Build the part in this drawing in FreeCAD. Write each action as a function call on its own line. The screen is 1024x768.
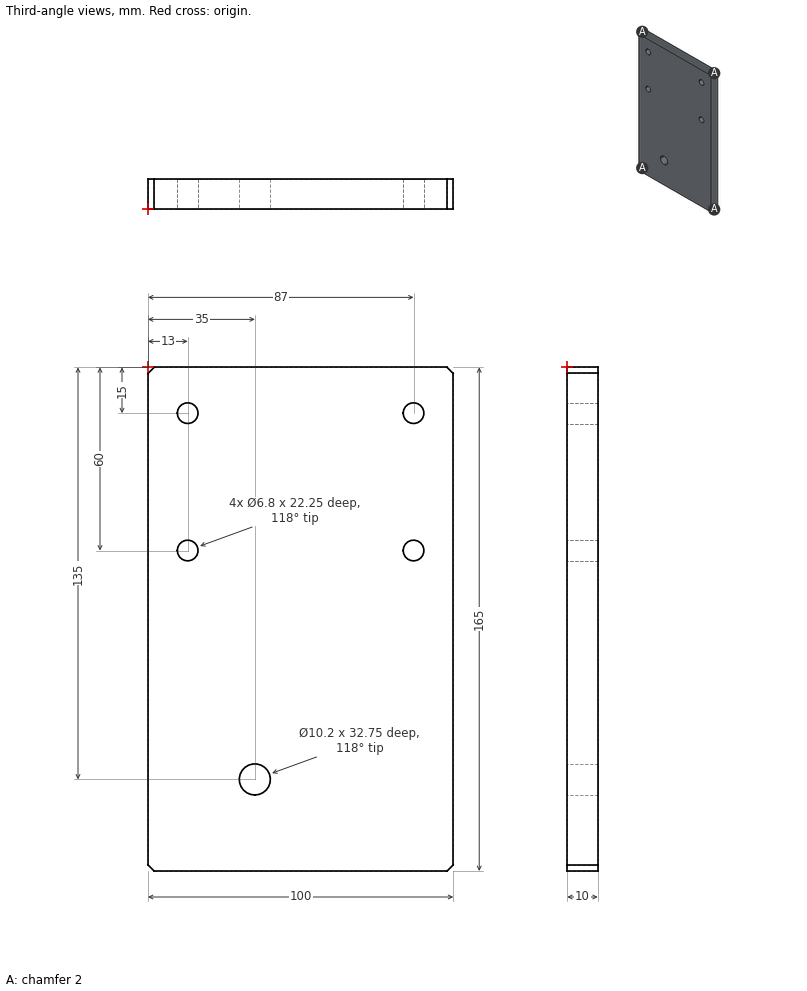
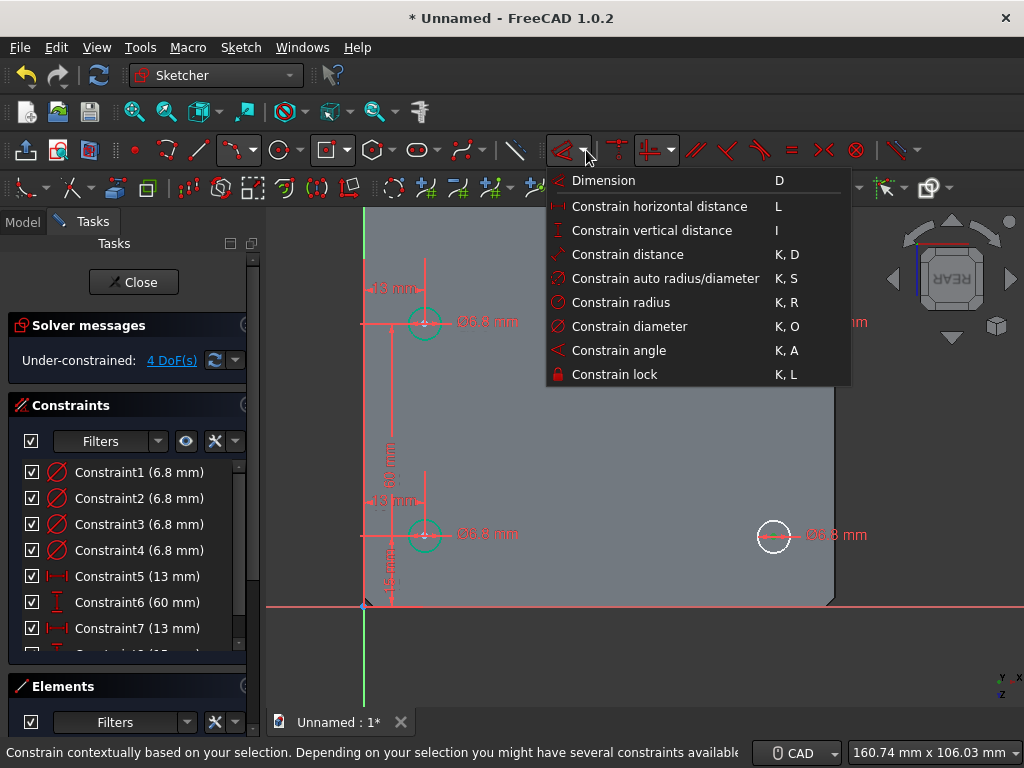
click(699, 206)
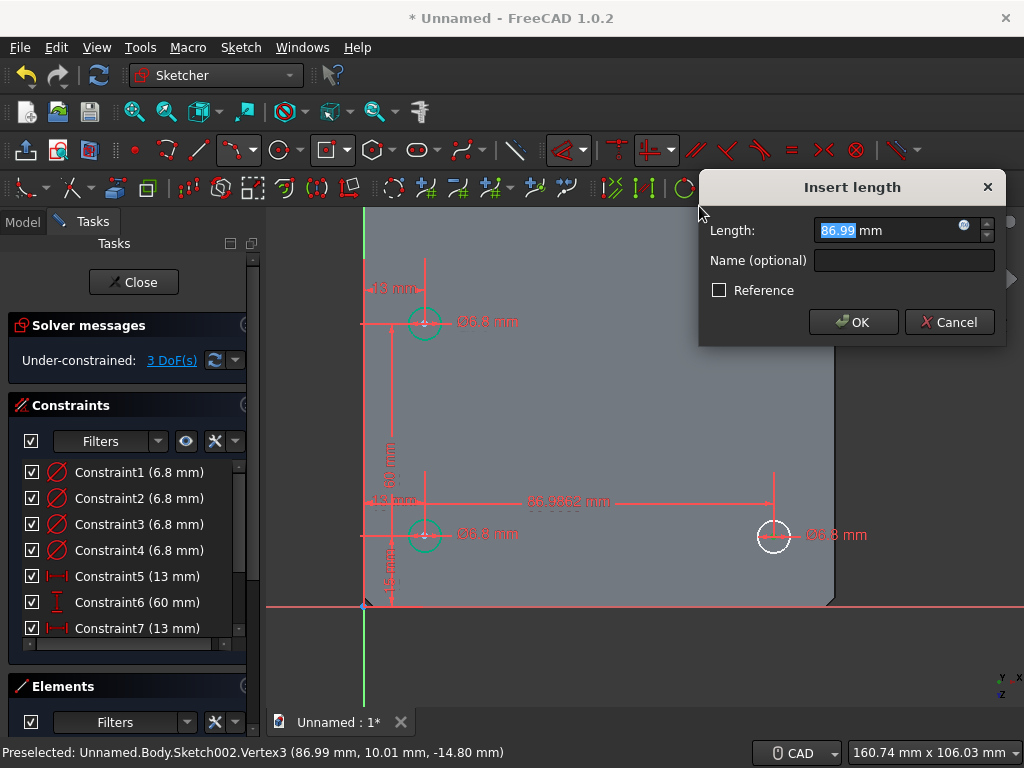
text(87)
key(Return)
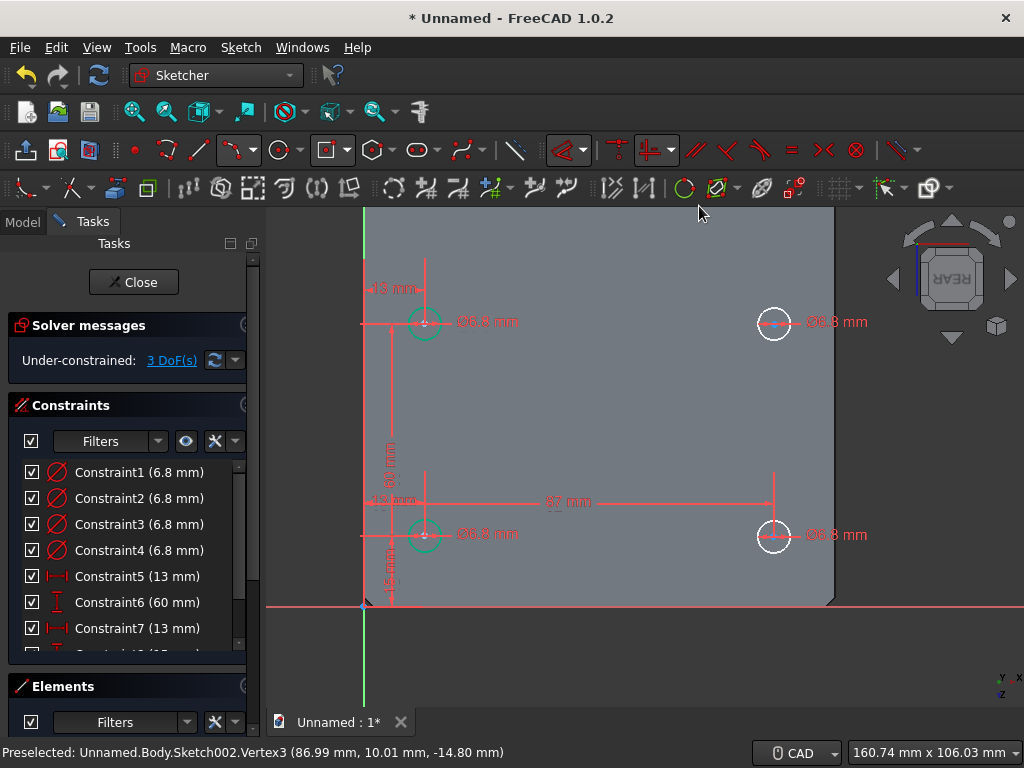
click(774, 537)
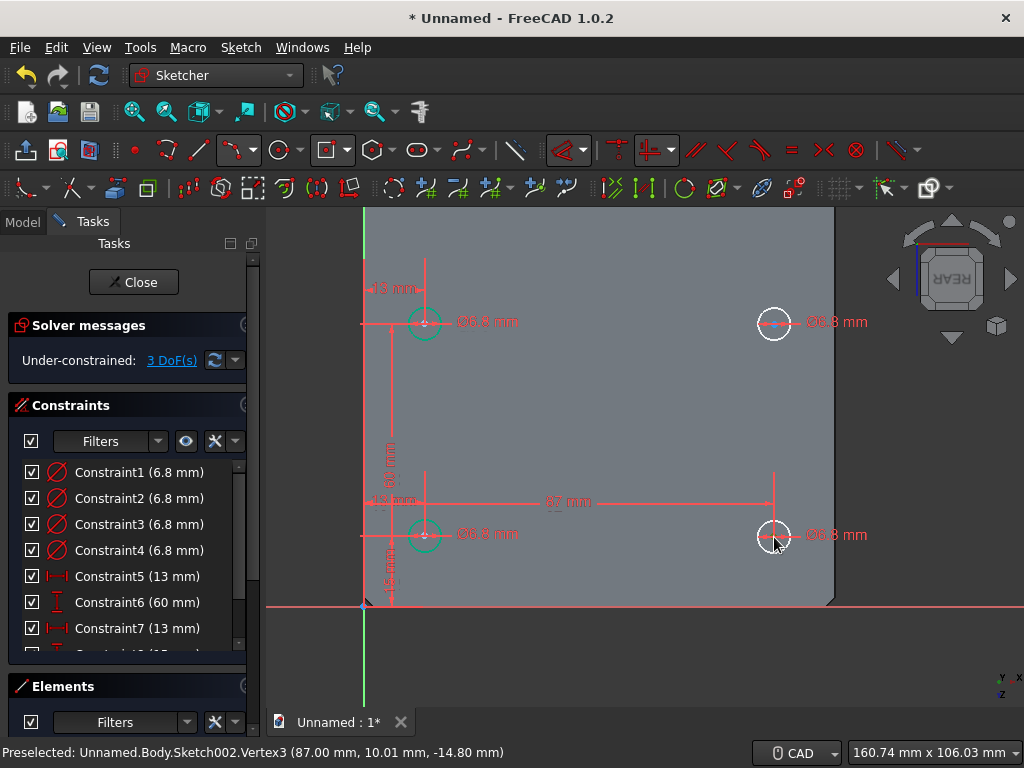
key(i)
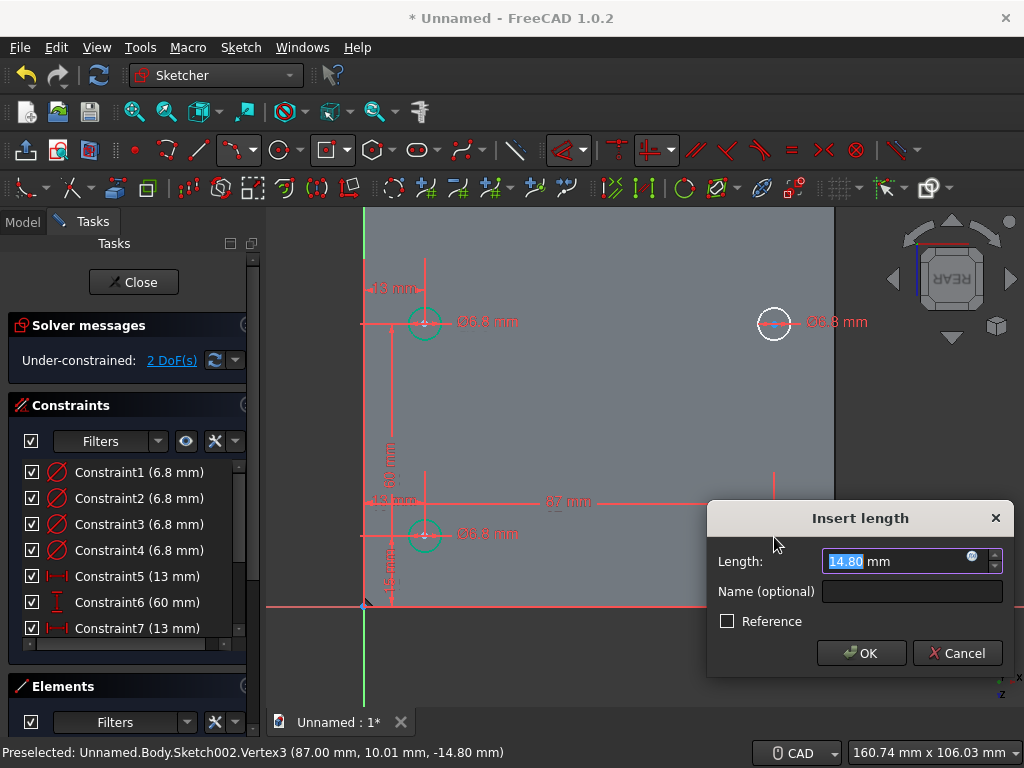
text(15)
key(Return)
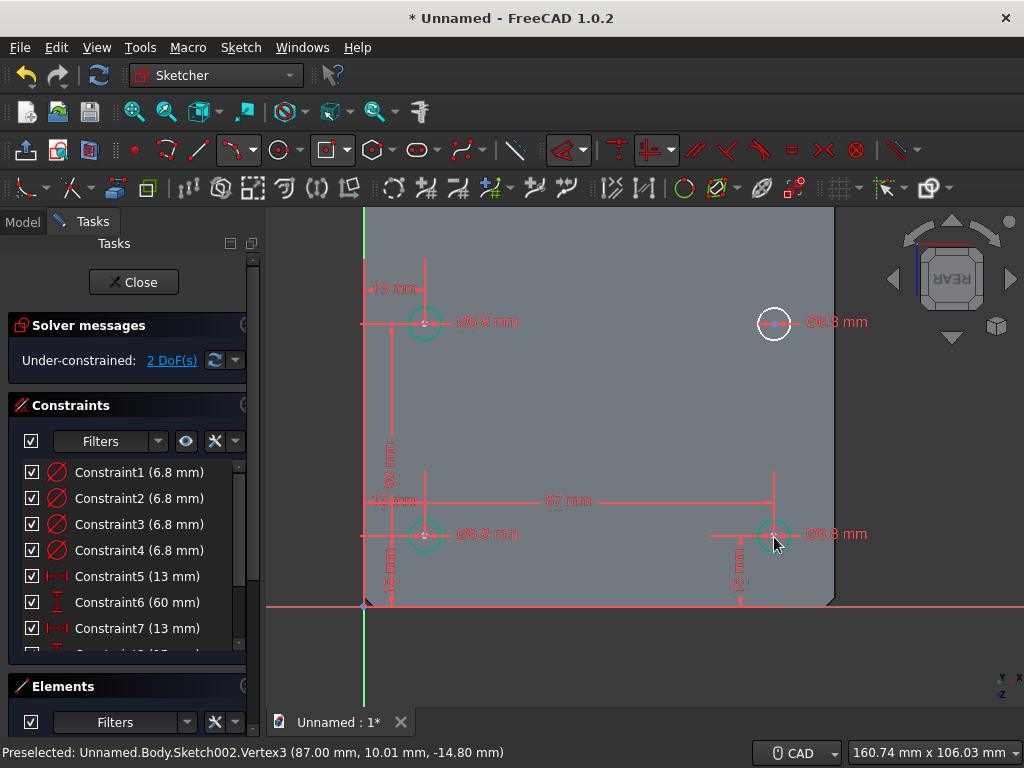
click(774, 324)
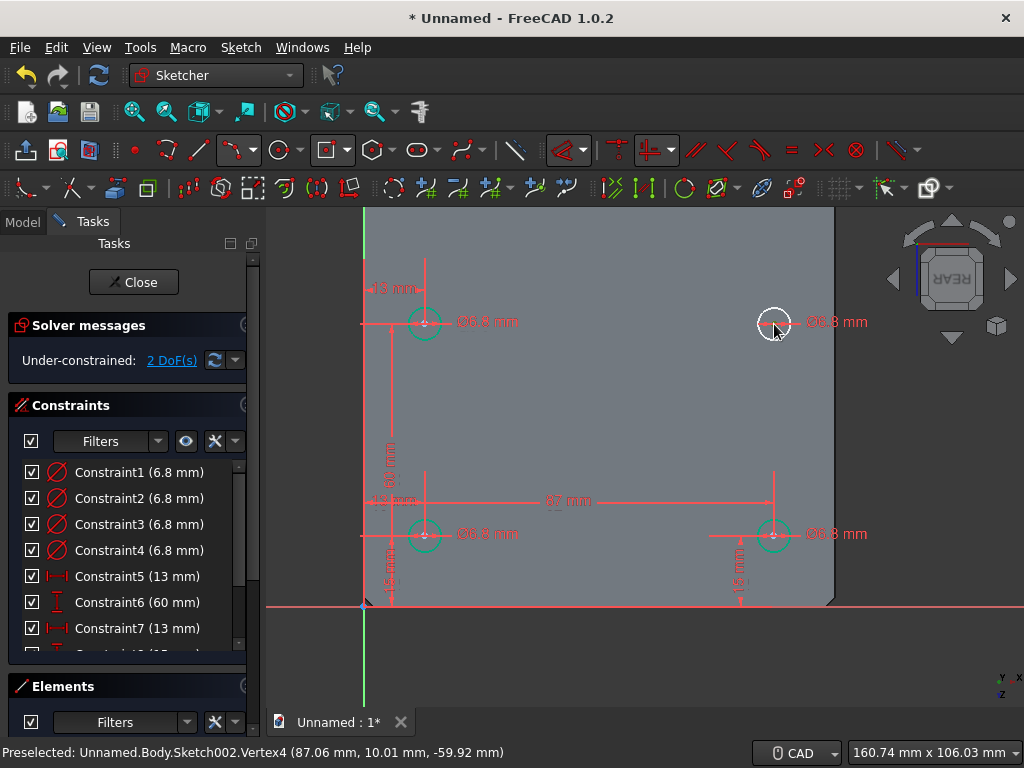
key(l)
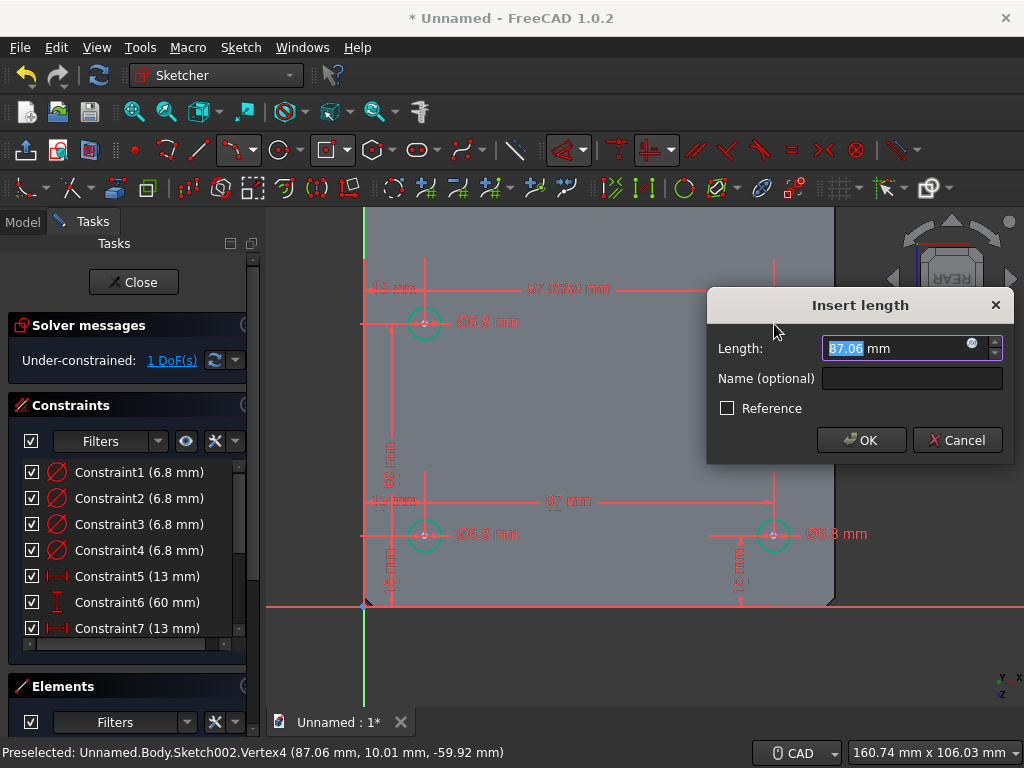
text(87)
key(Return)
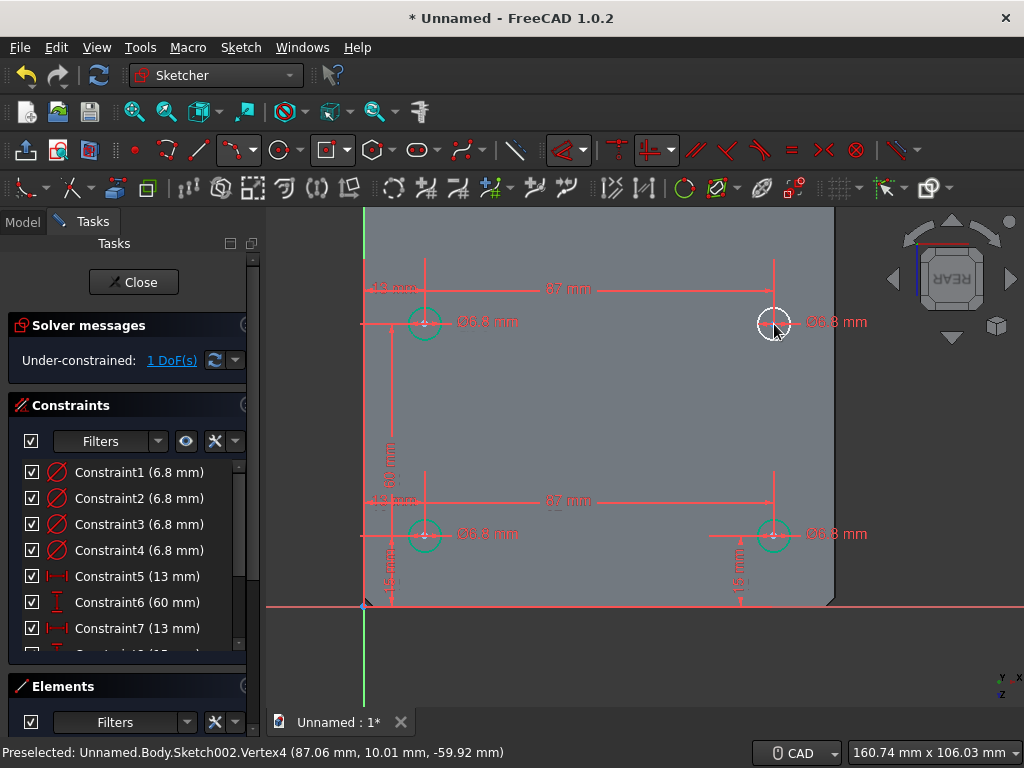
click(774, 324)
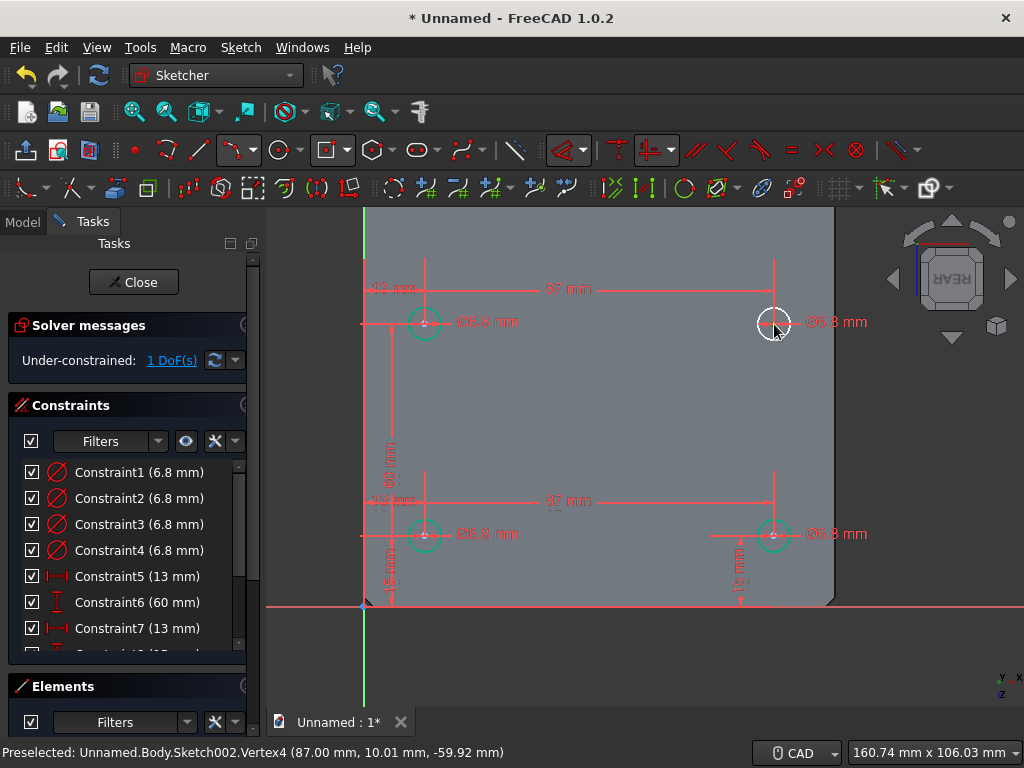
key(i)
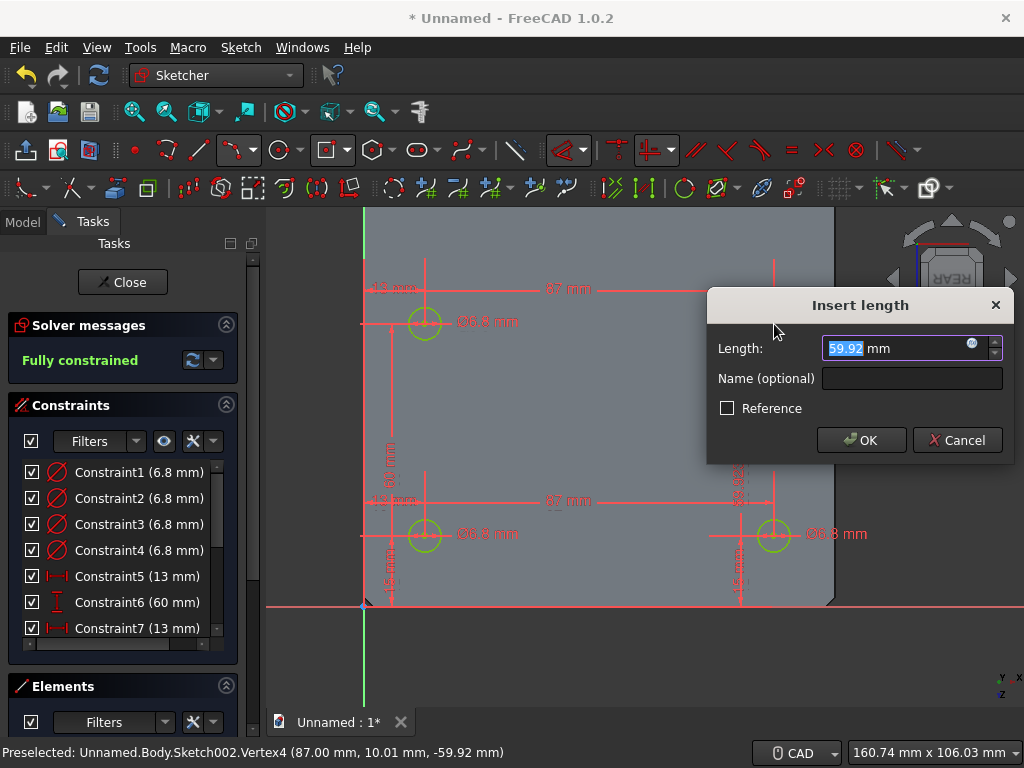
text(60)
key(Return)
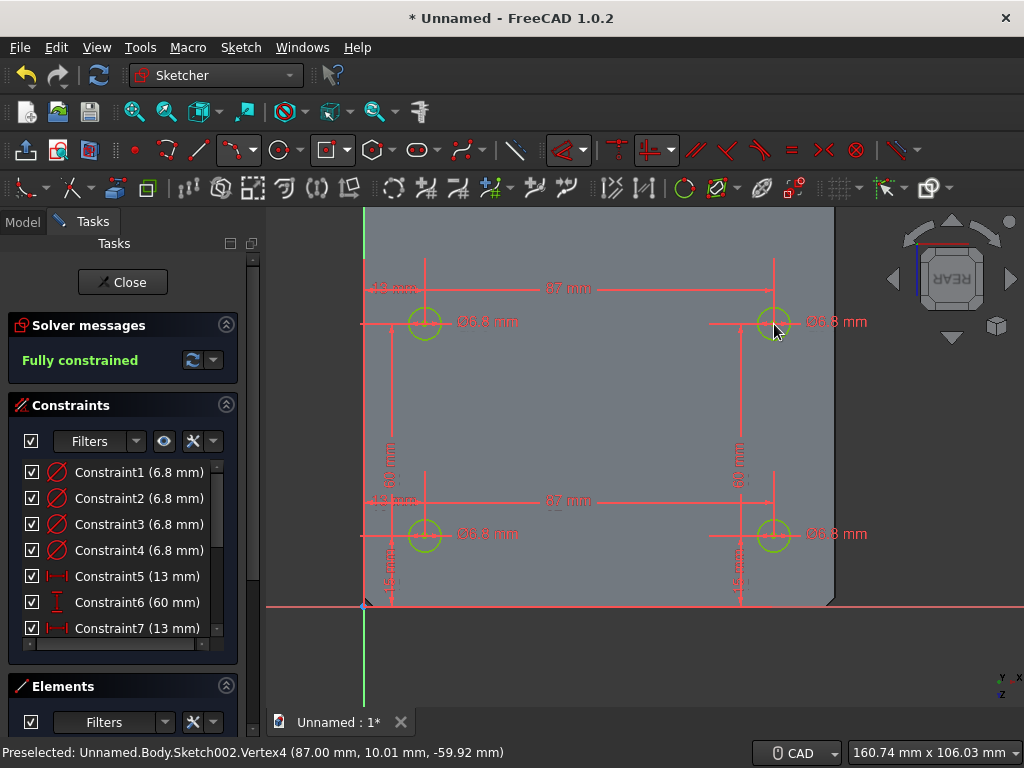
click(123, 282)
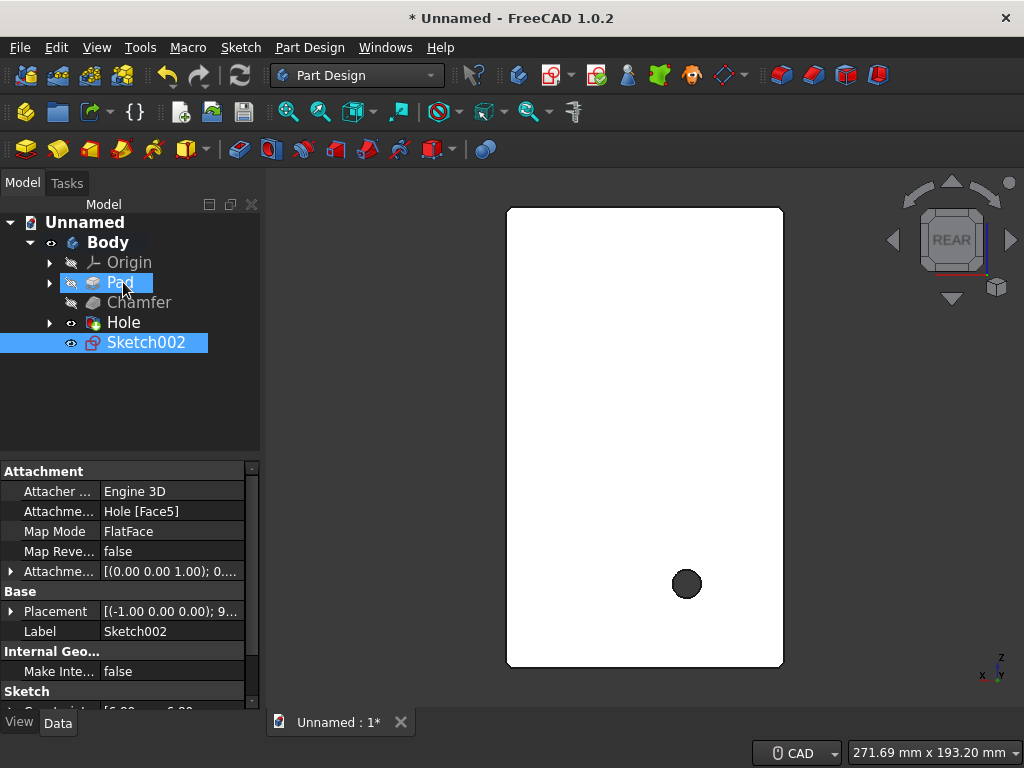
click(272, 150)